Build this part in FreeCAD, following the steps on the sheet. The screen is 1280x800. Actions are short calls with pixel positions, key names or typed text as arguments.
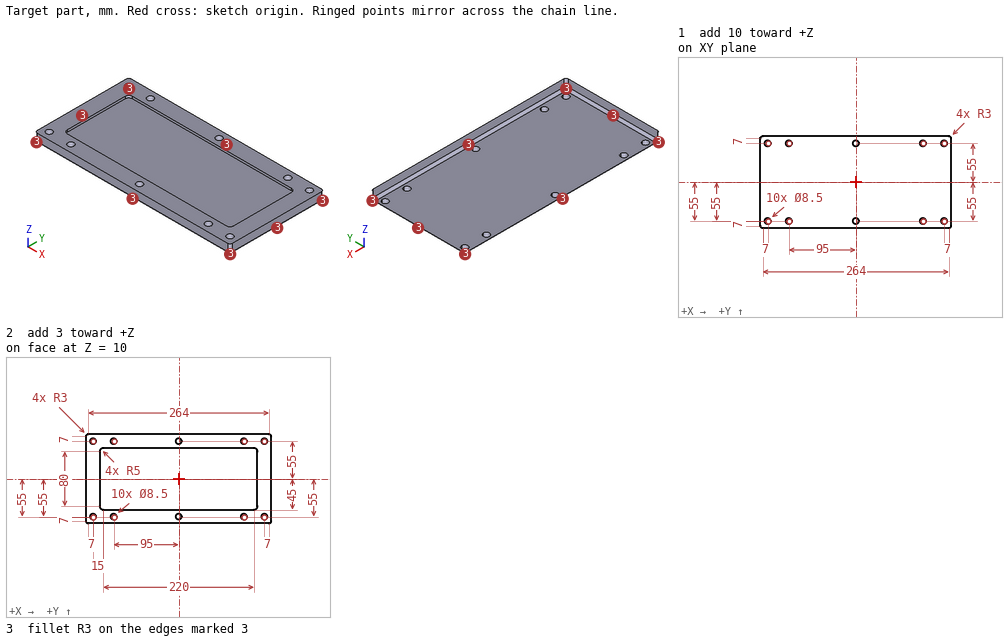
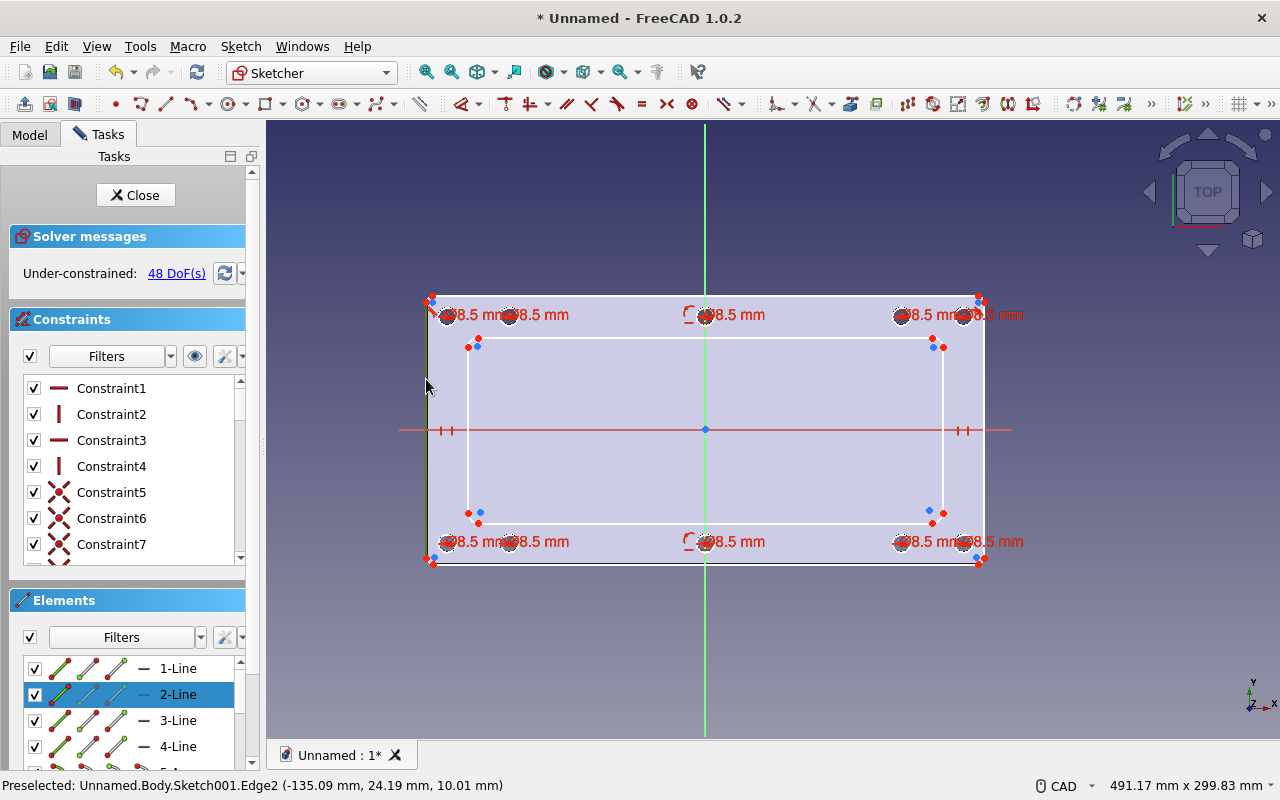
scroll(428, 298, up, 6)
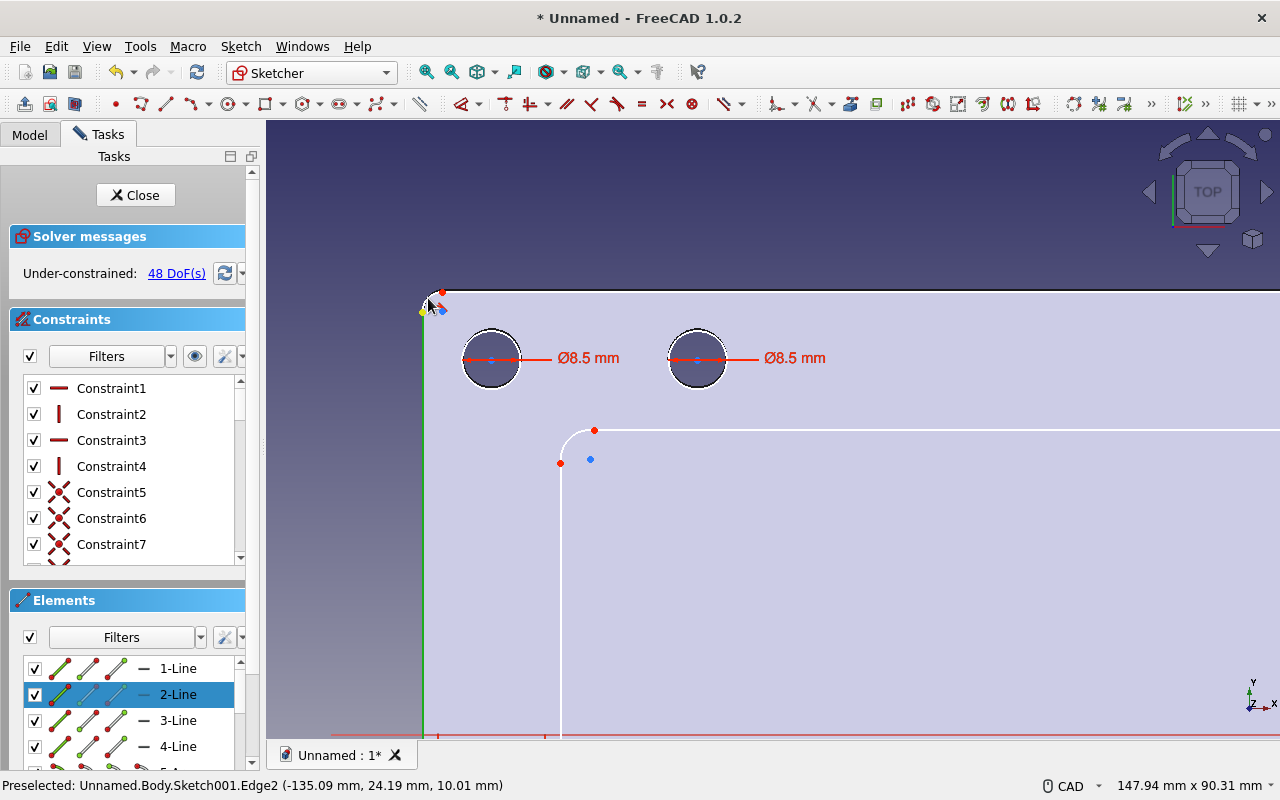
click(428, 298)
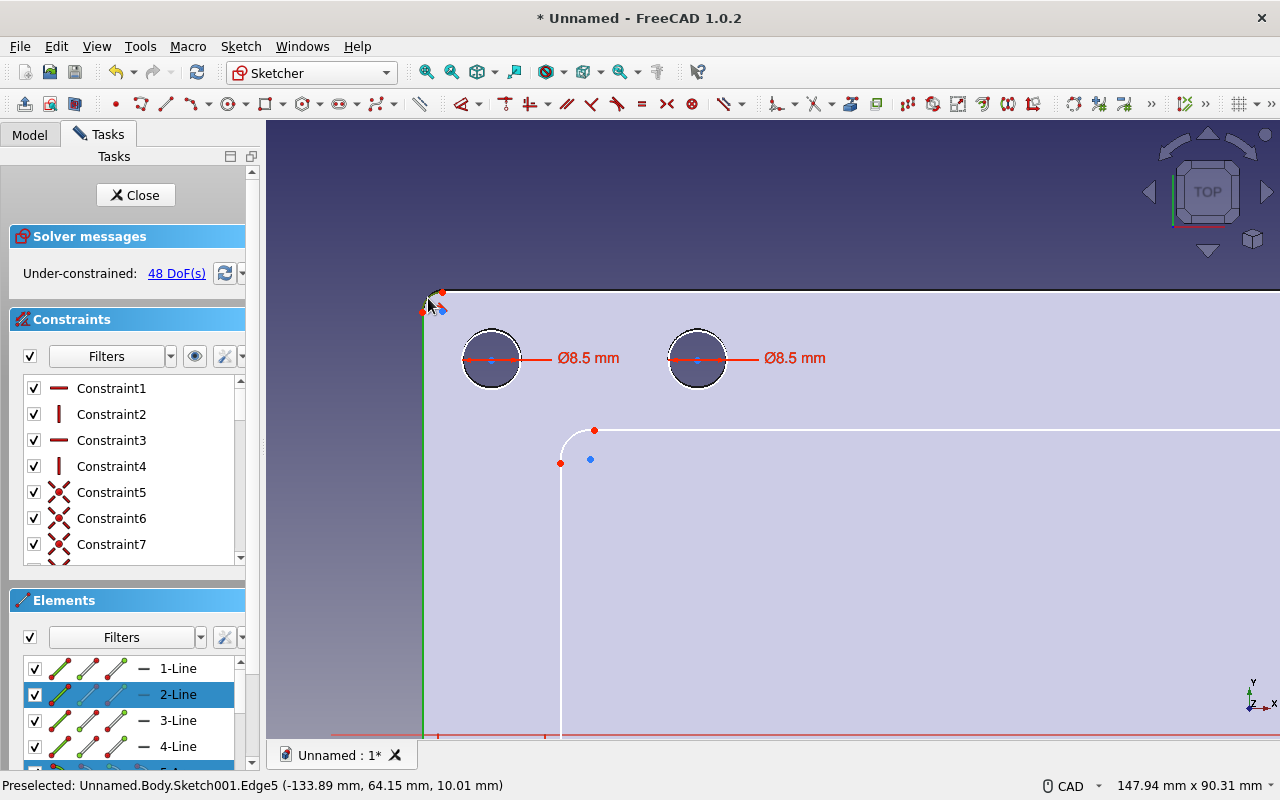
click(617, 104)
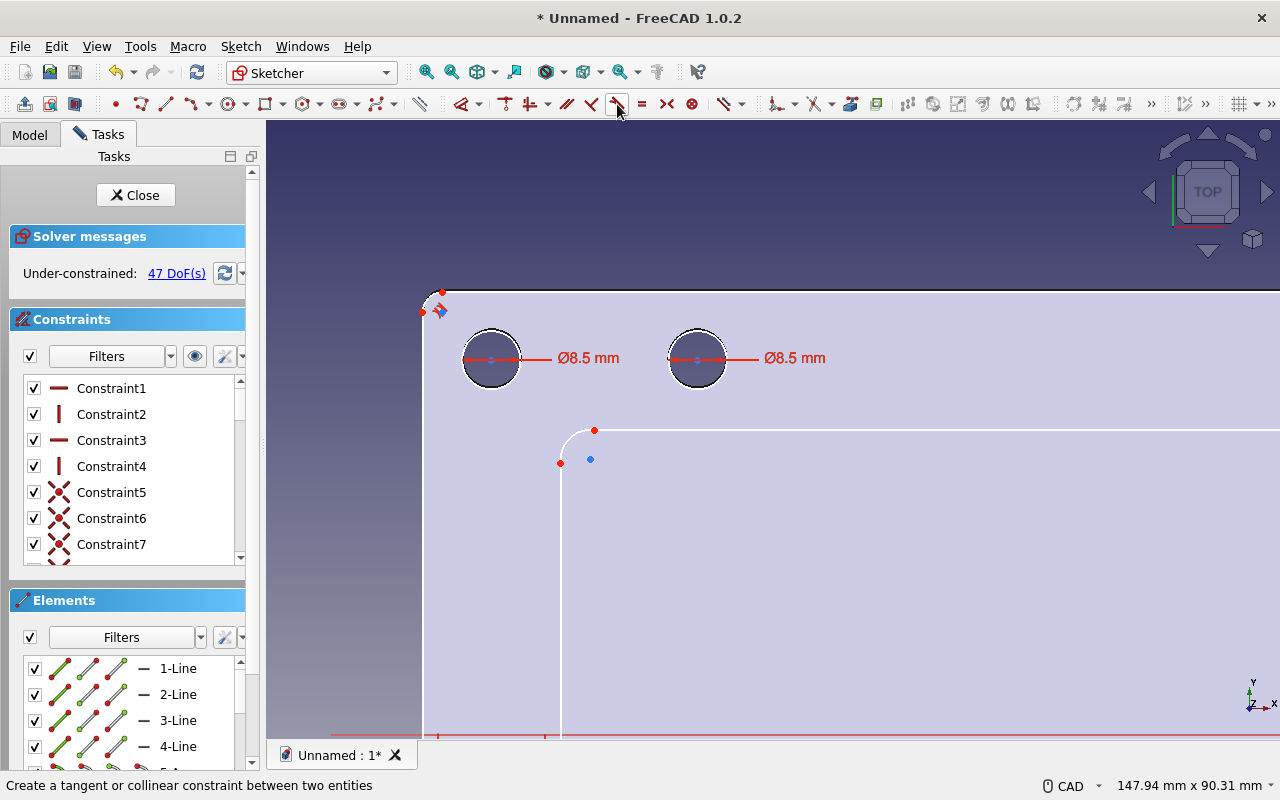
click(423, 567)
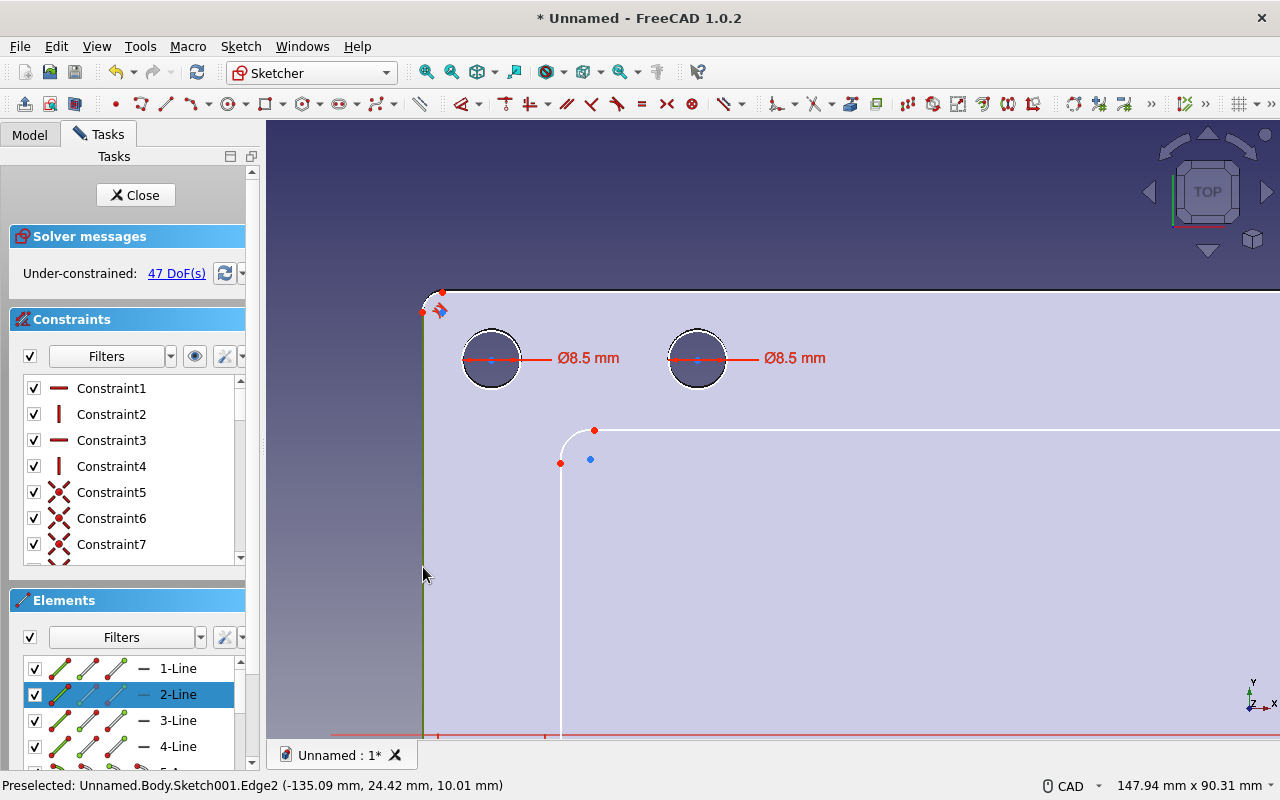
scroll(427, 298, down, 6)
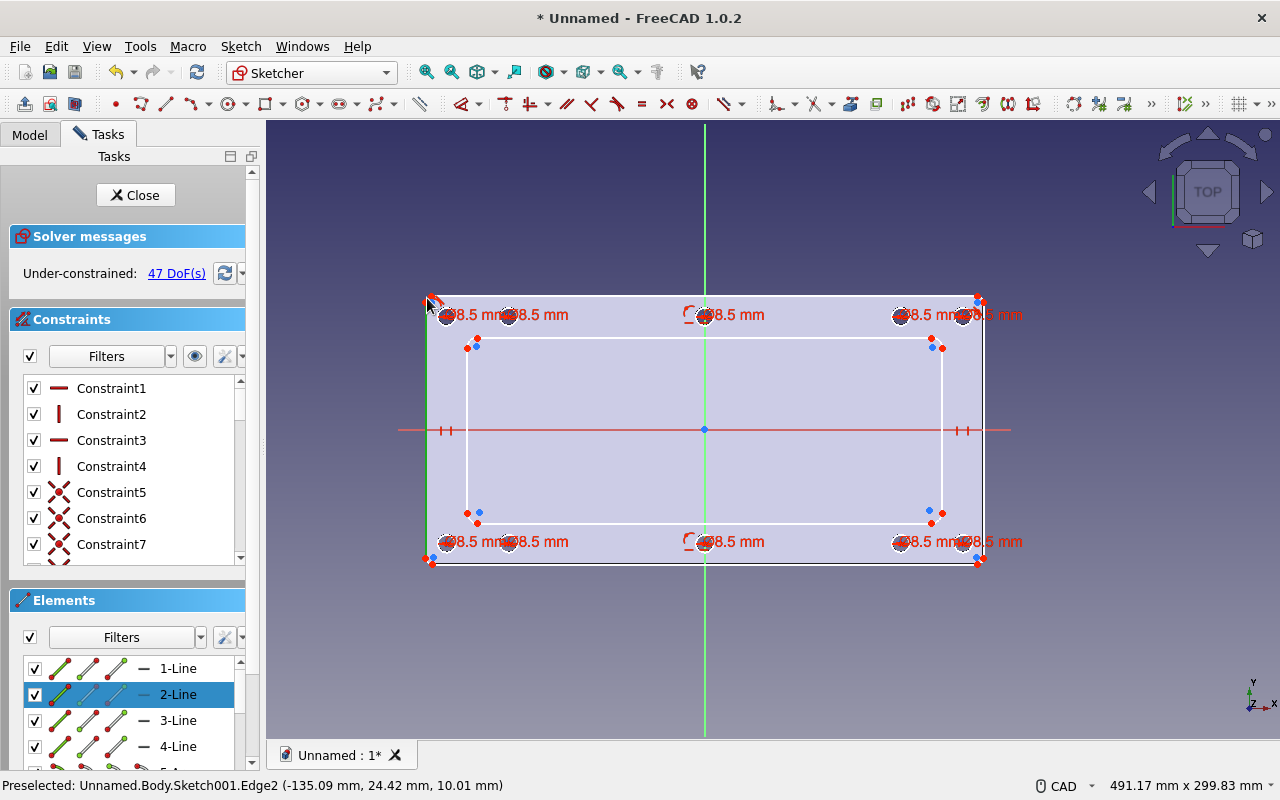
scroll(427, 561, up, 8)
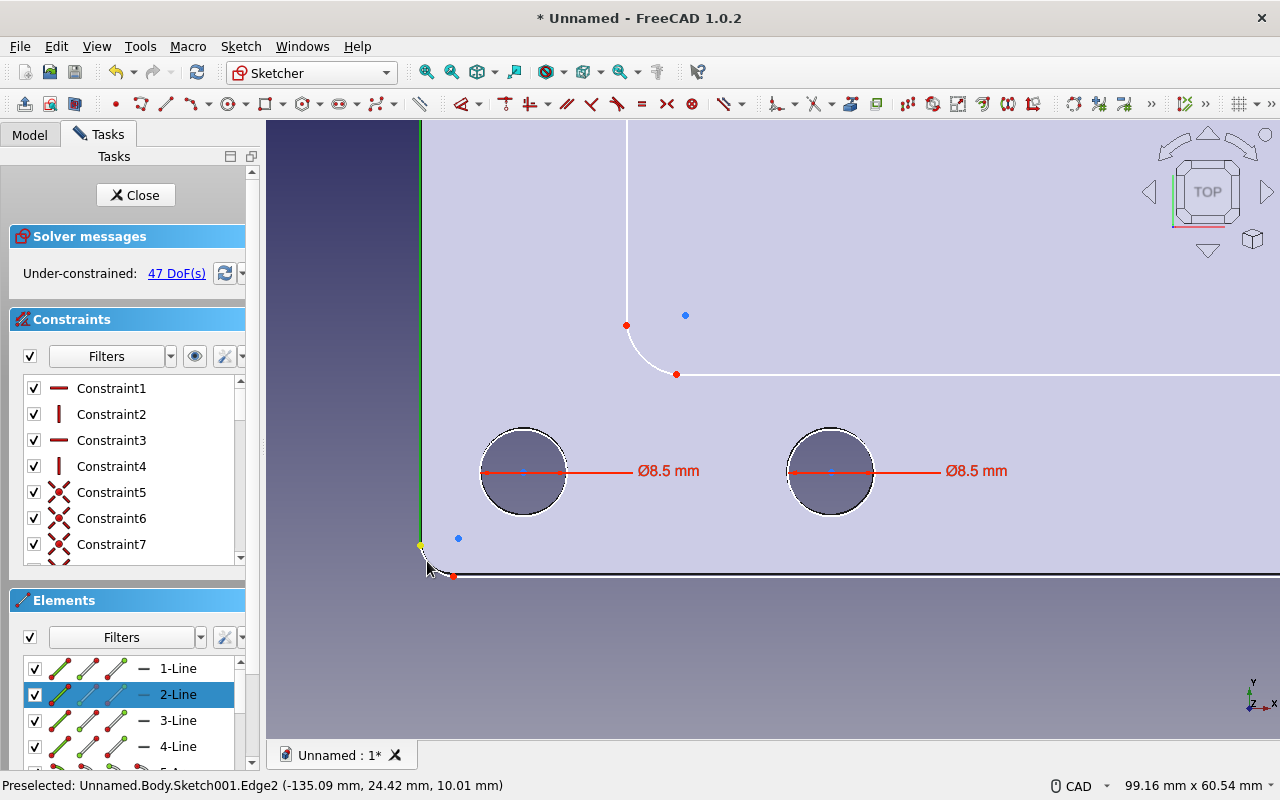
click(426, 559)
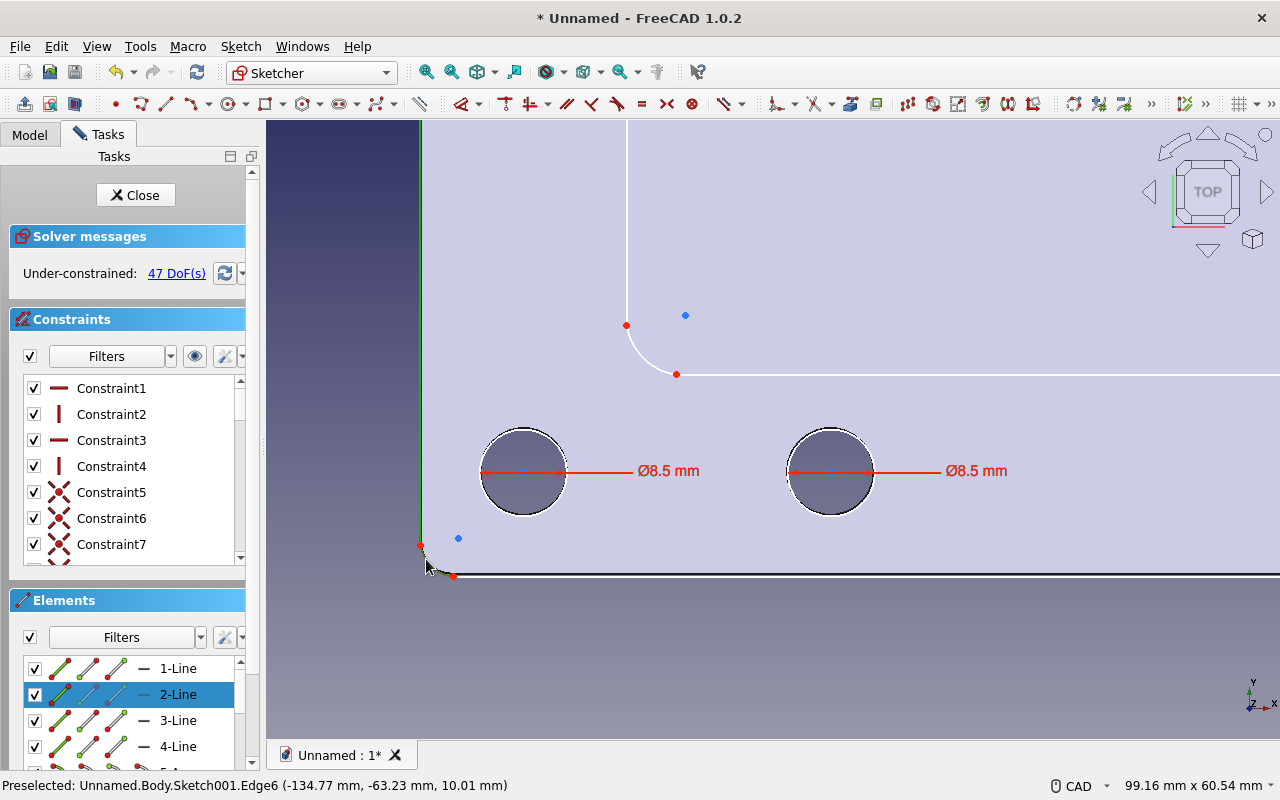
click(617, 104)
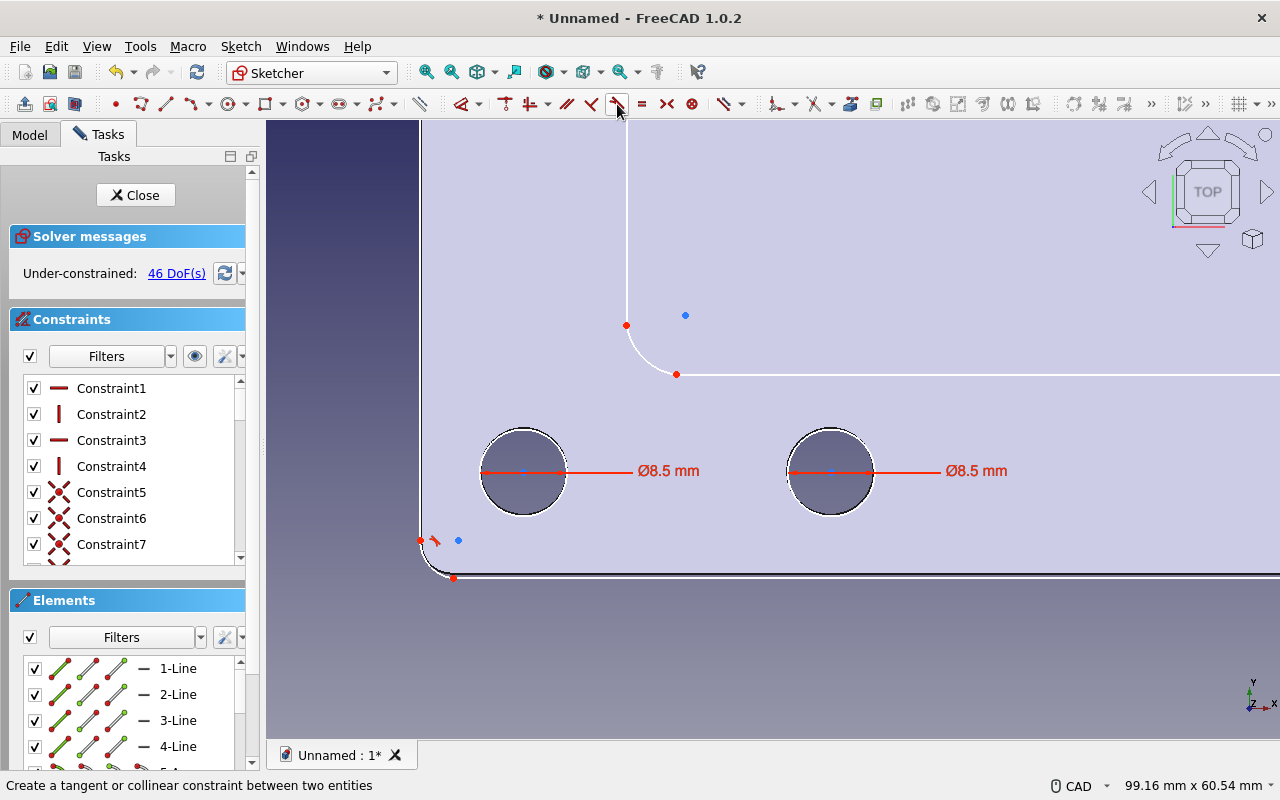
scroll(427, 561, down, 8)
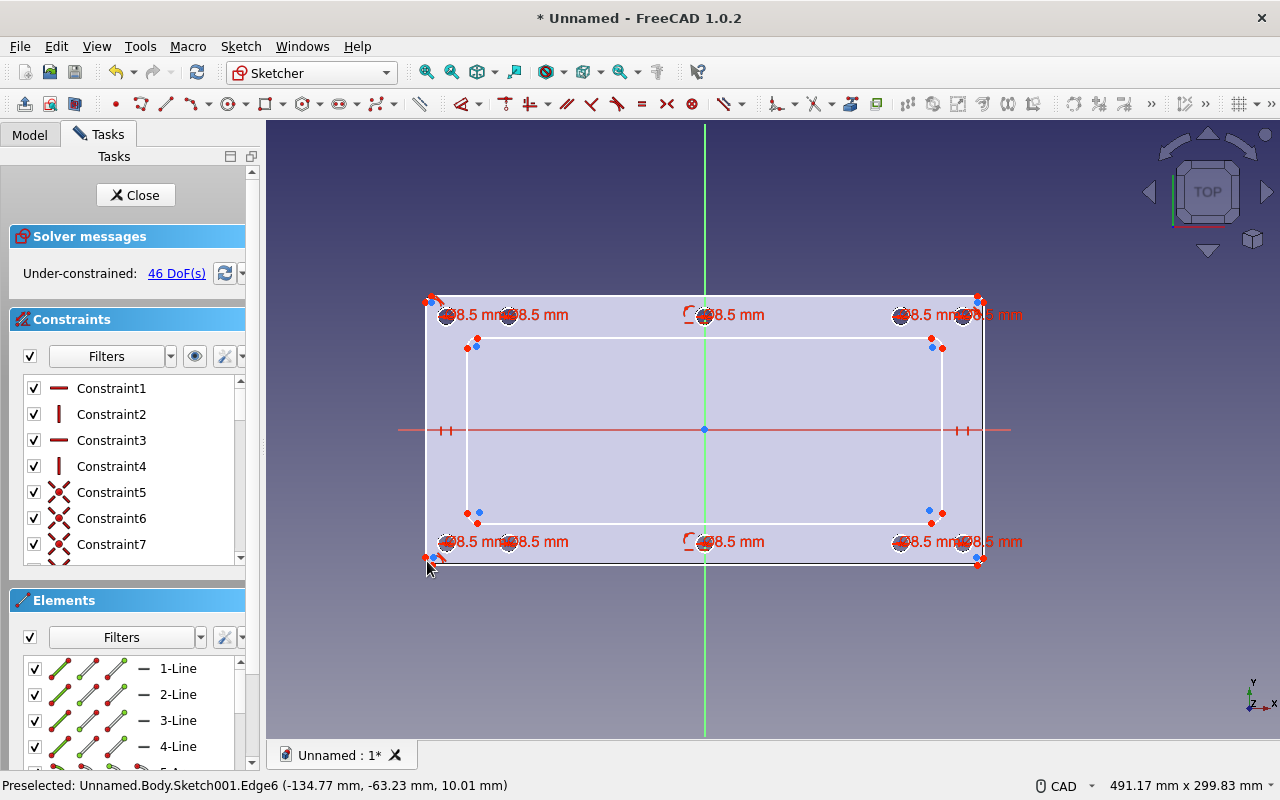
click(541, 565)